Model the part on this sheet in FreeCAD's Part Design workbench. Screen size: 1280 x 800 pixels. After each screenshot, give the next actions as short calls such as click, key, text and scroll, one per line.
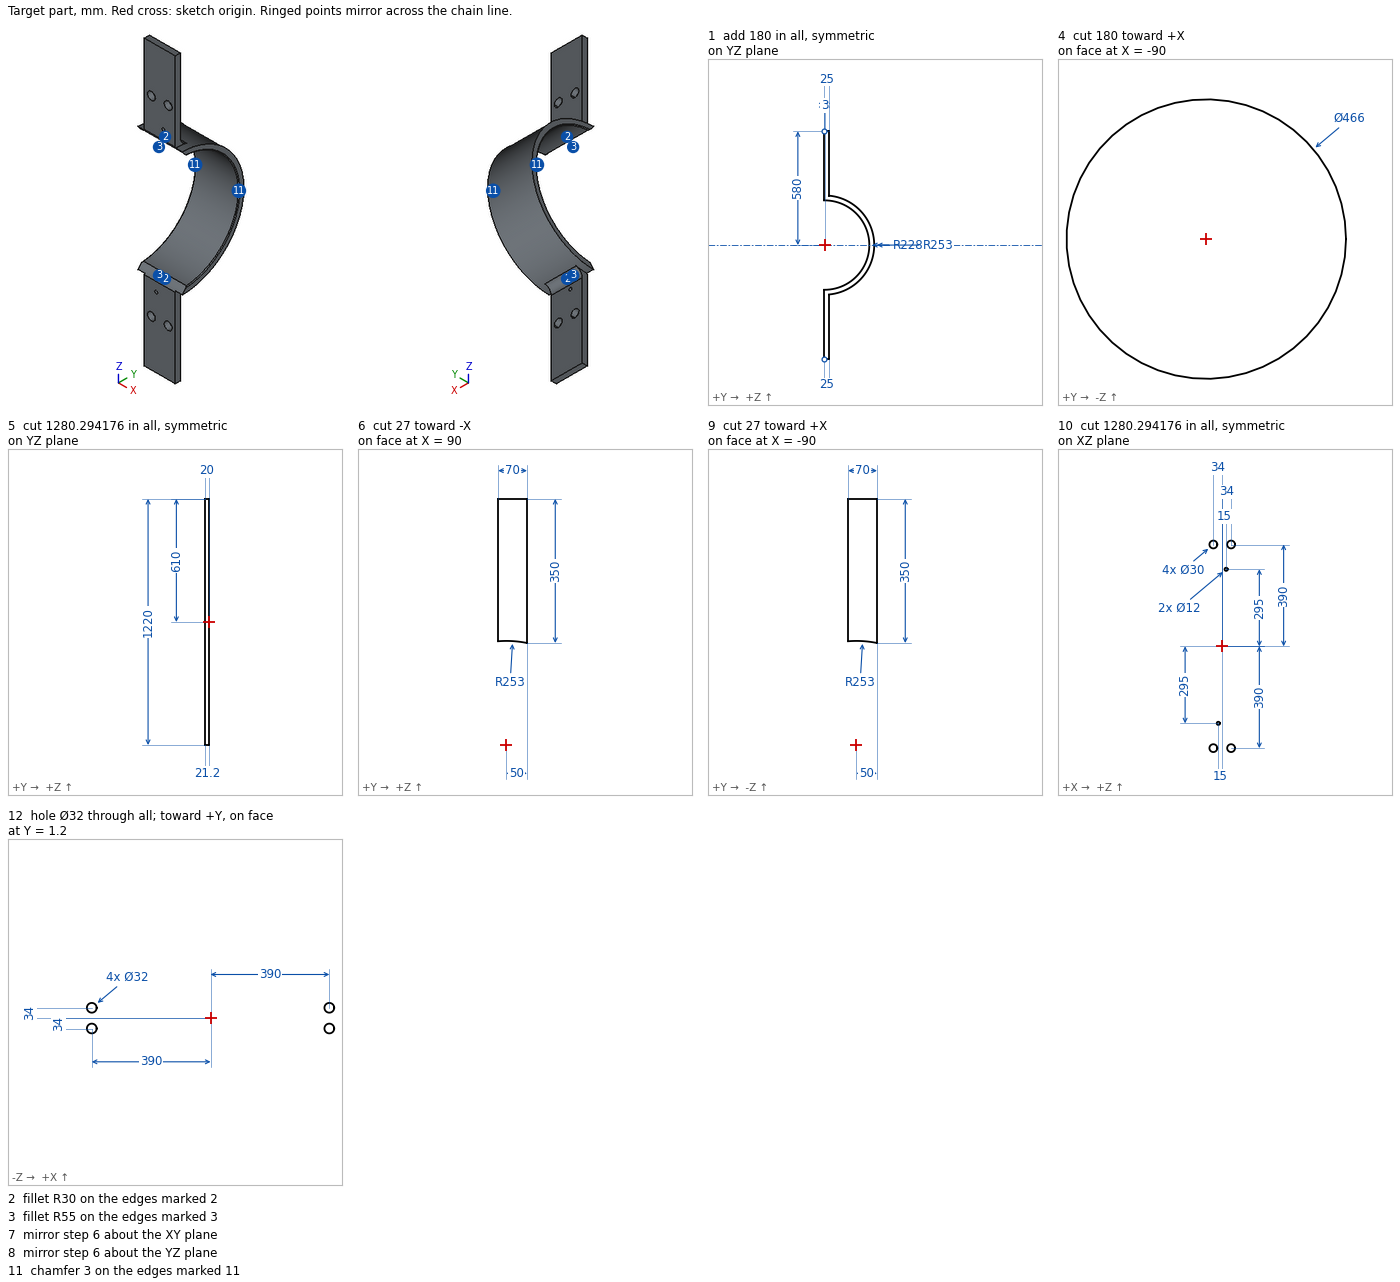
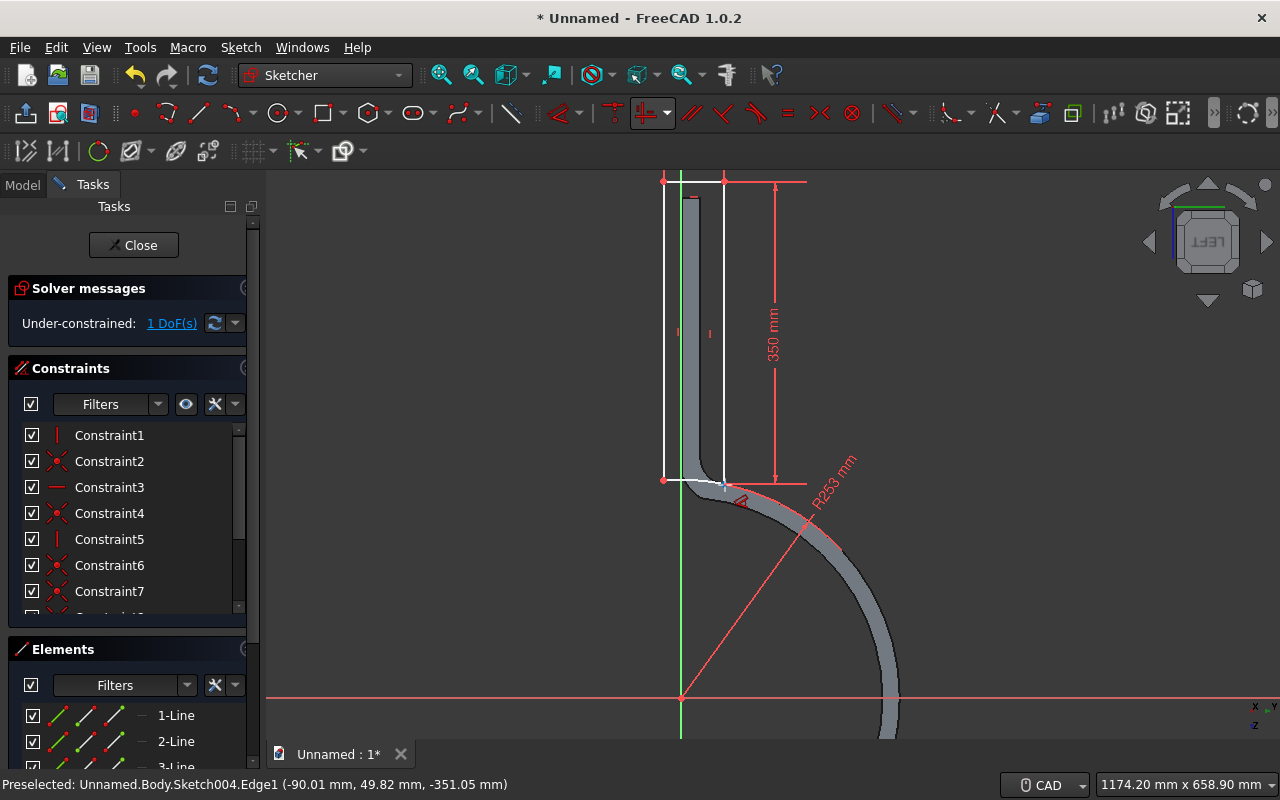
click(724, 484)
click(703, 450)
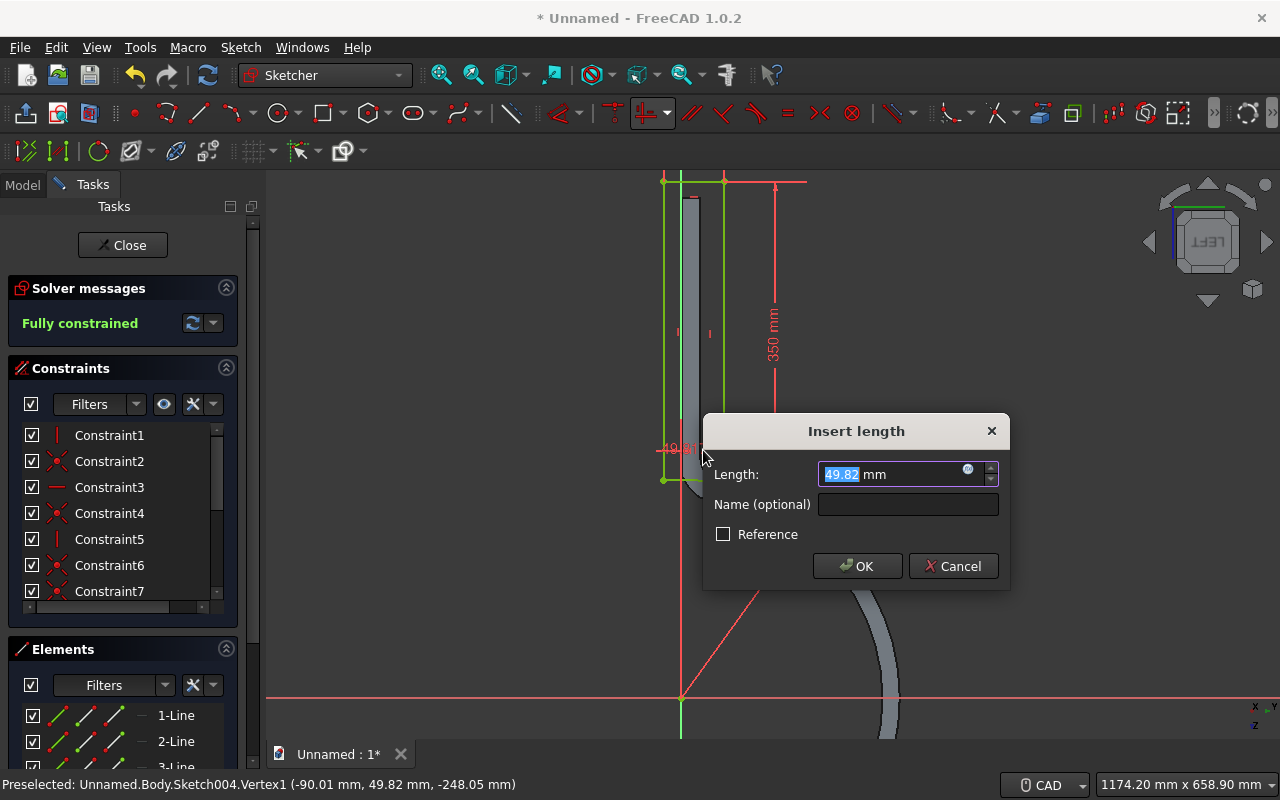
text(50)
key(Return)
key(Escape)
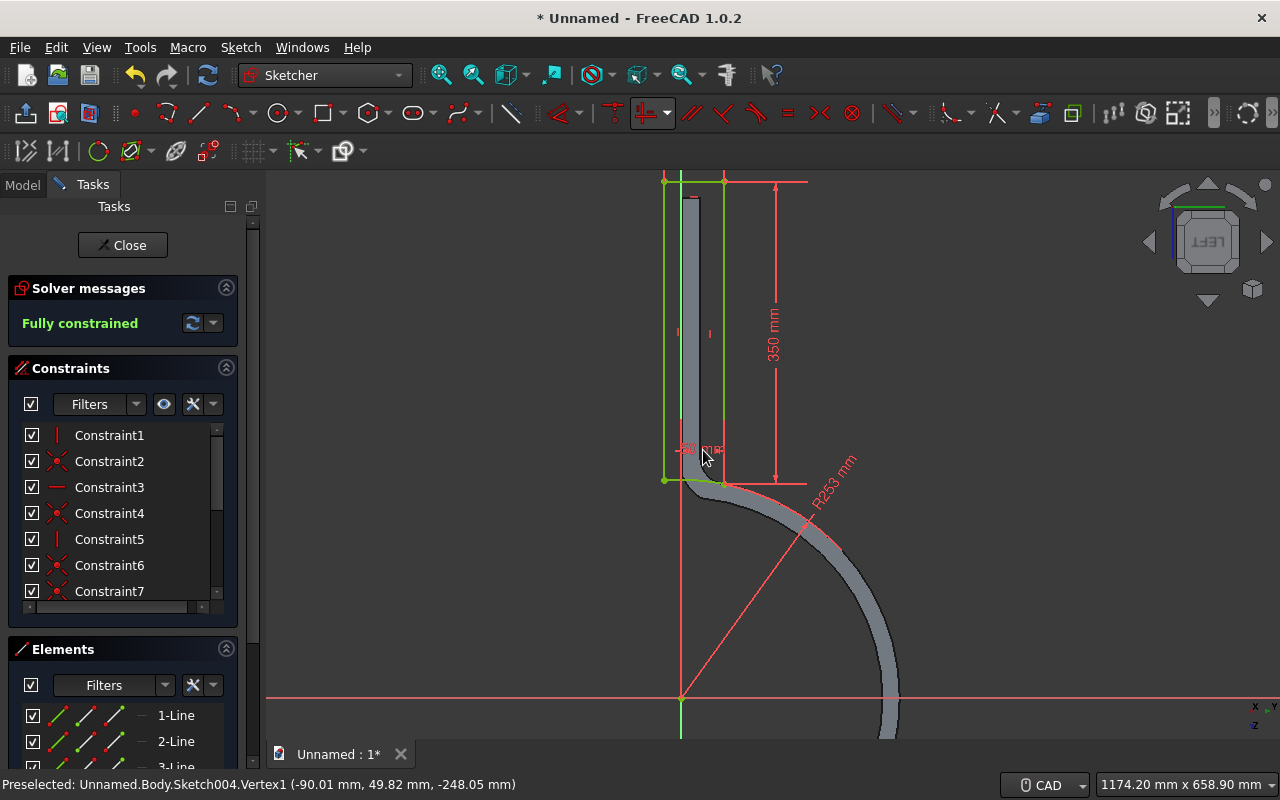
click(123, 245)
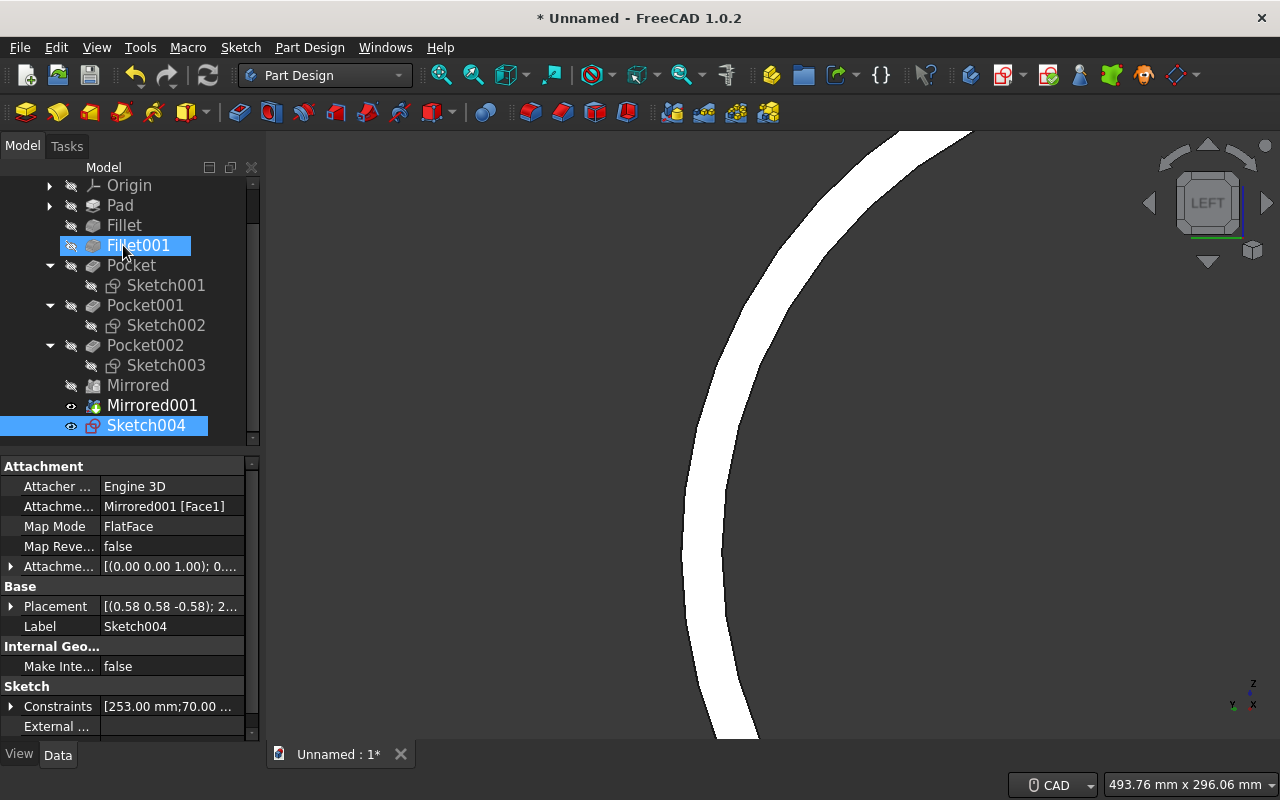
click(240, 112)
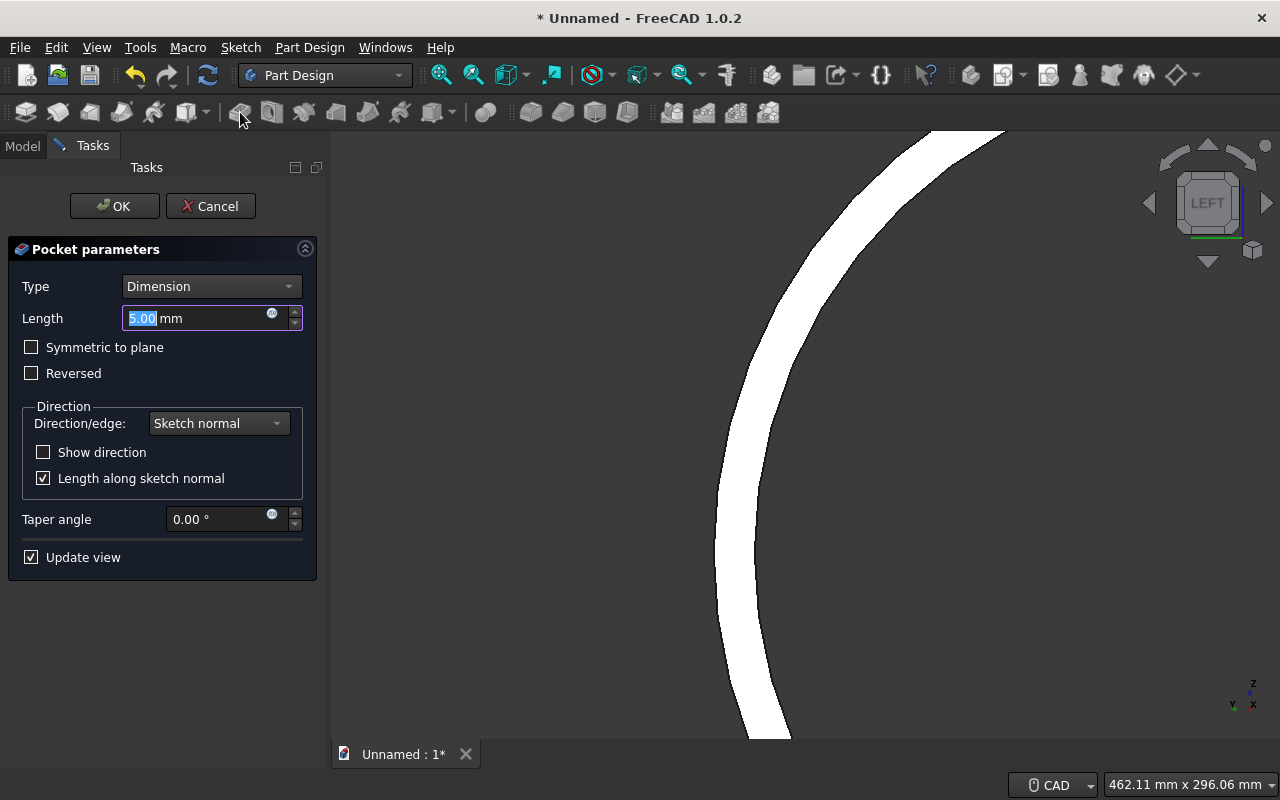
text(27)
key(Tab)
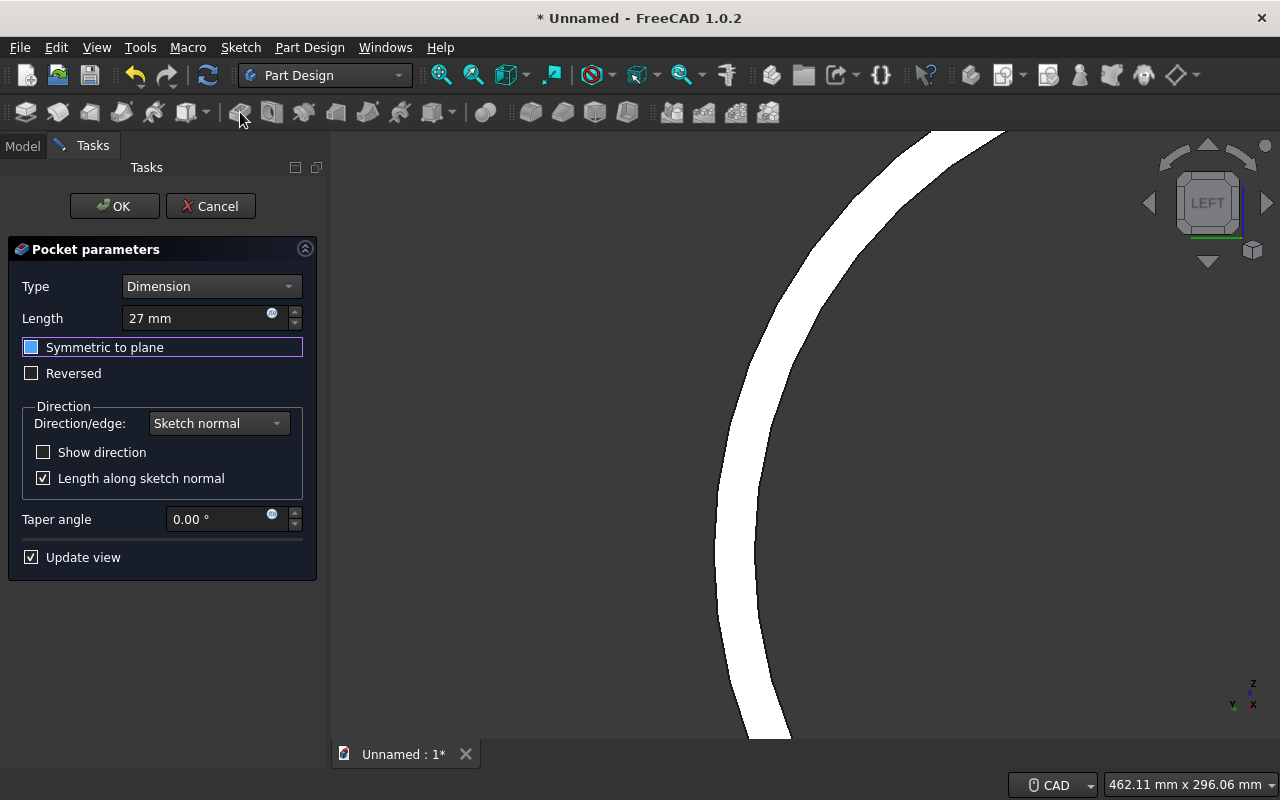
click(115, 206)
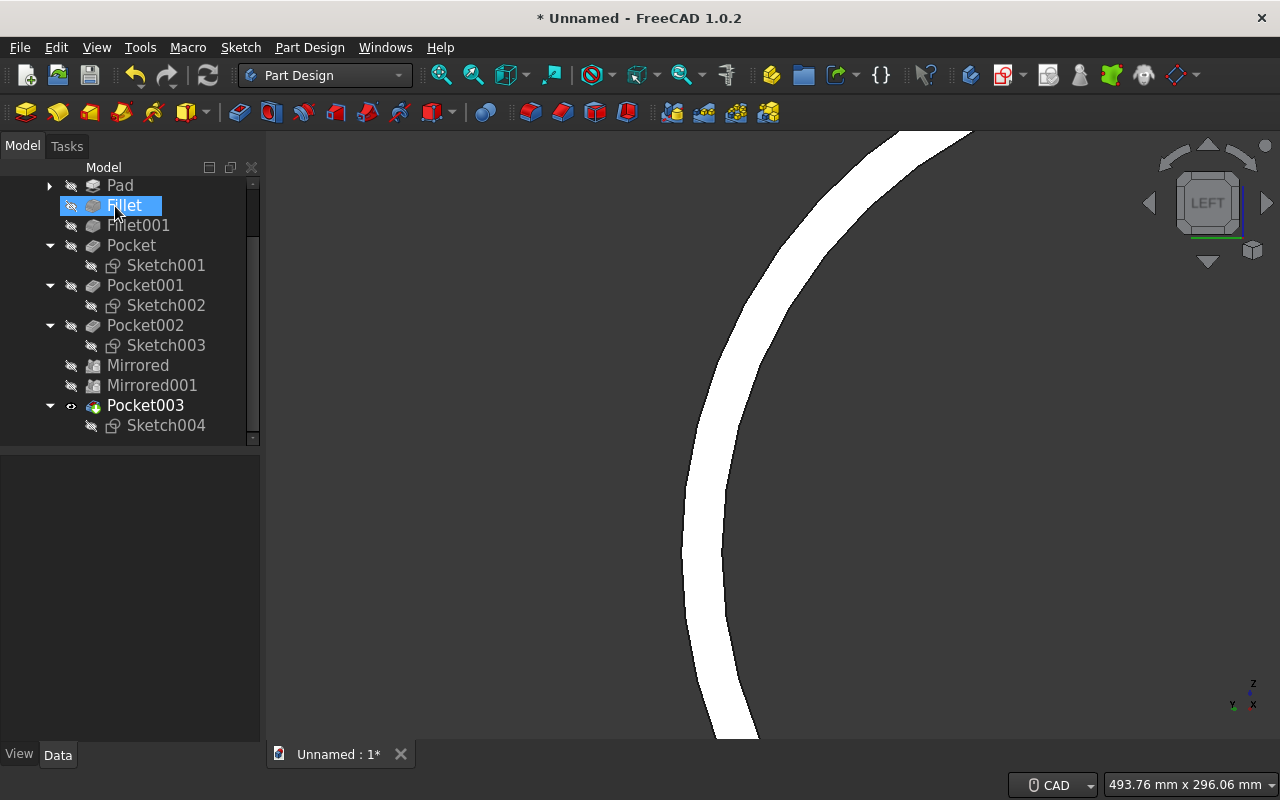
click(442, 76)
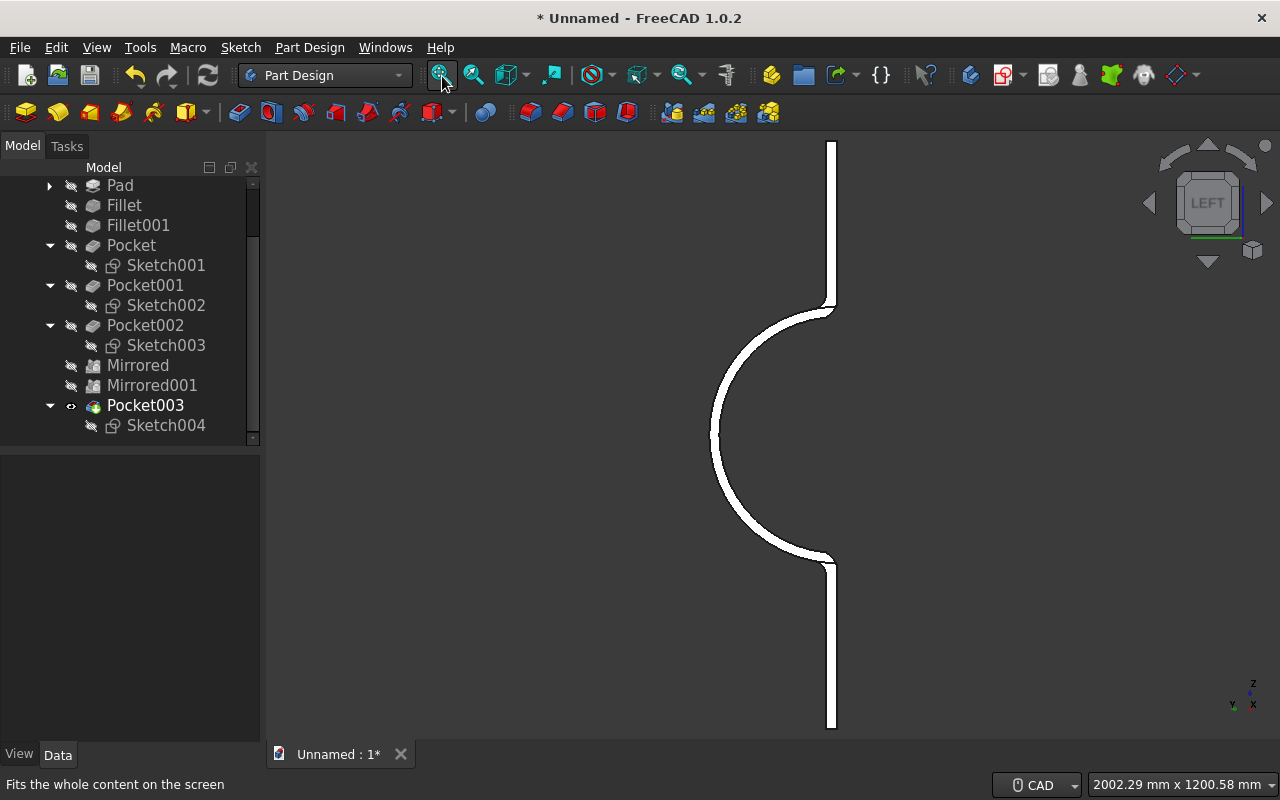
click(1004, 76)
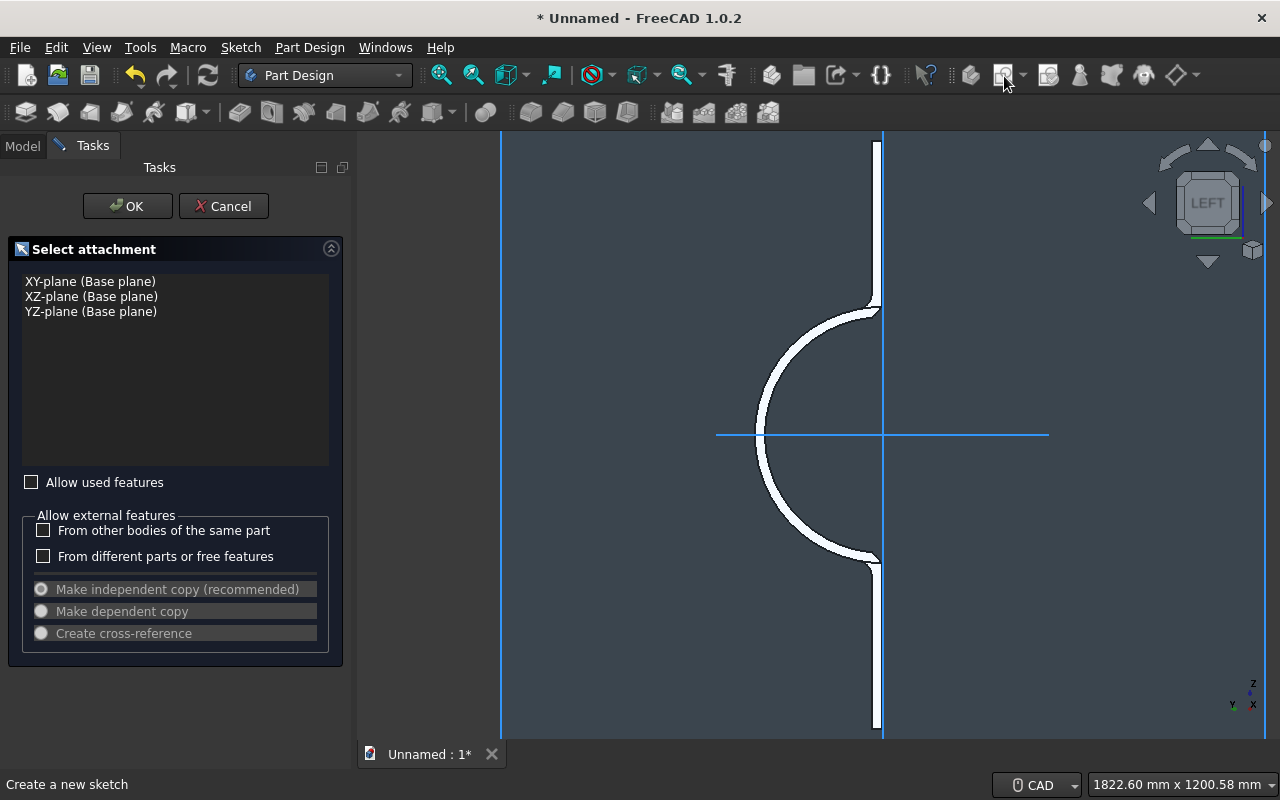
click(82, 296)